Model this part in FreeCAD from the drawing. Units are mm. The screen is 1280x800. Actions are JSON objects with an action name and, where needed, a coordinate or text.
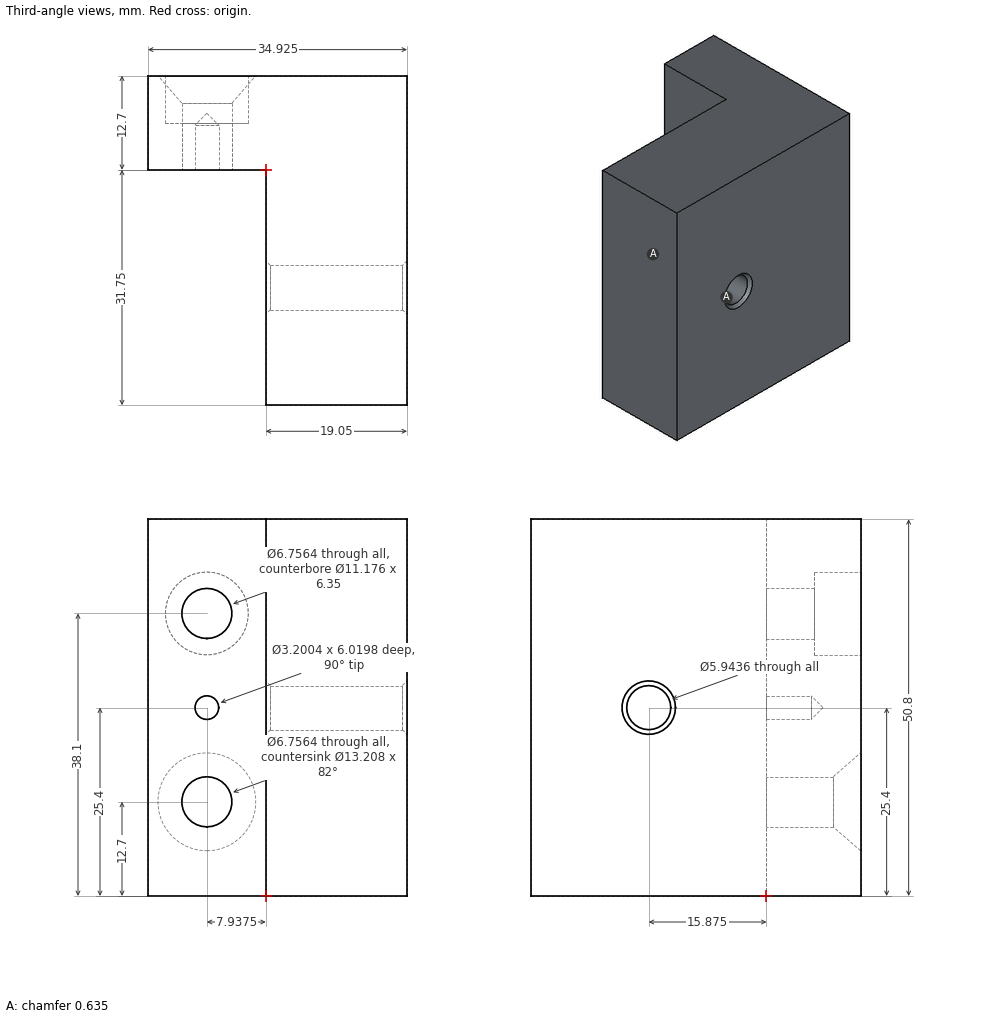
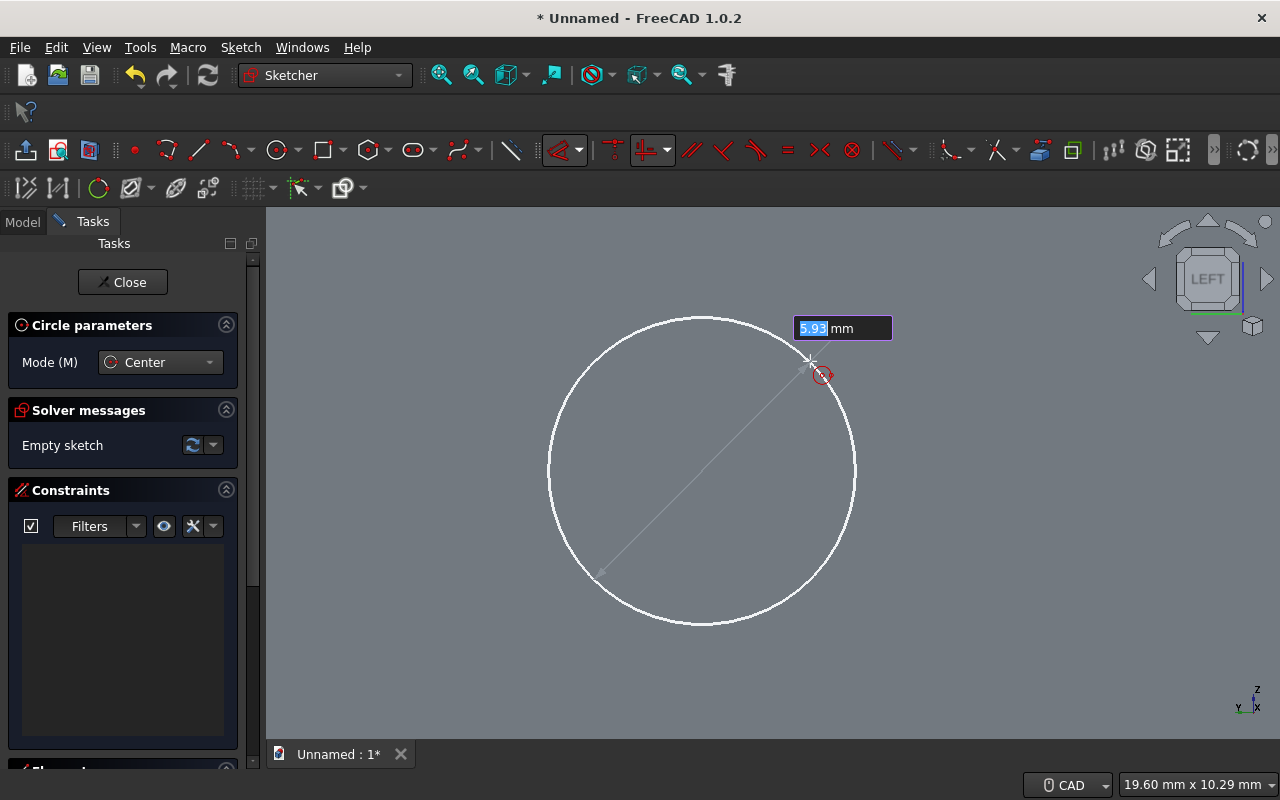
{"action": "type", "text": "5.9436"}
{"action": "key", "text": "Return"}
{"action": "key", "text": "Escape"}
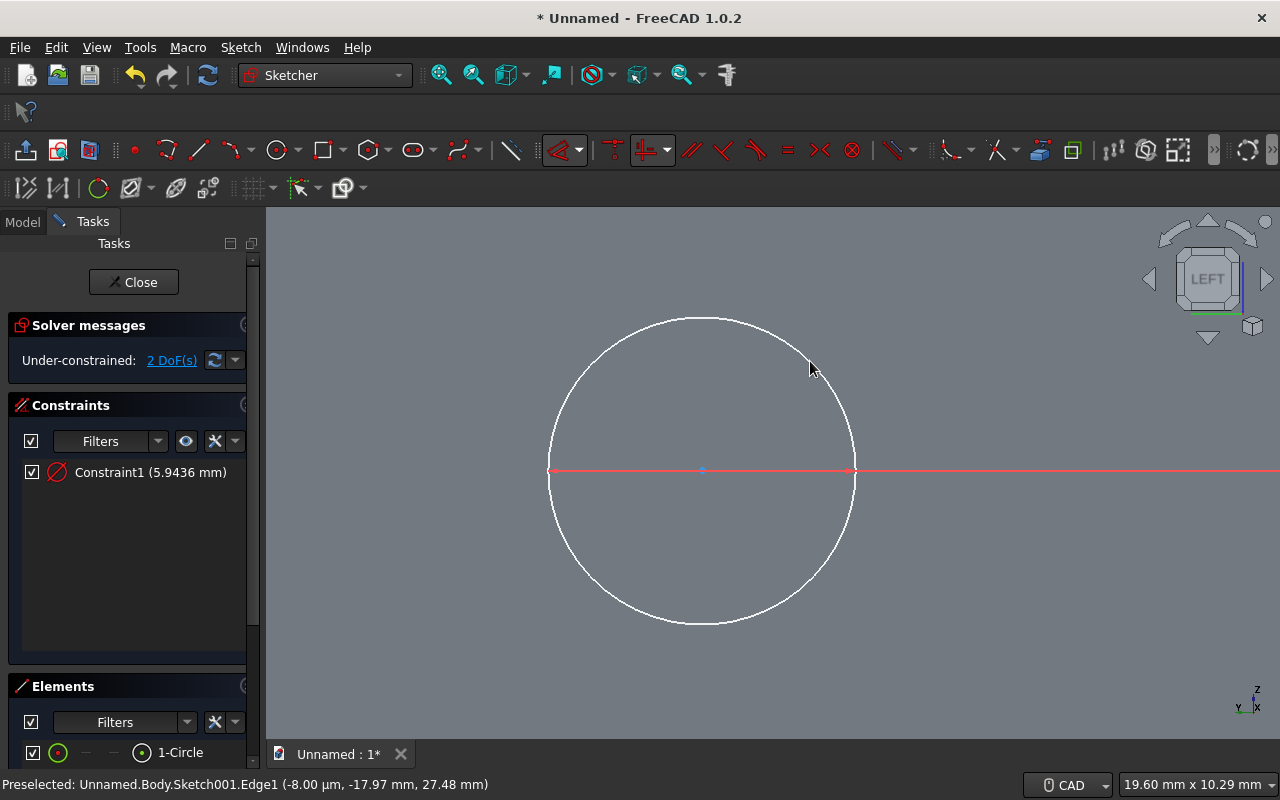
{"action": "left_click", "coordinate": [702, 471]}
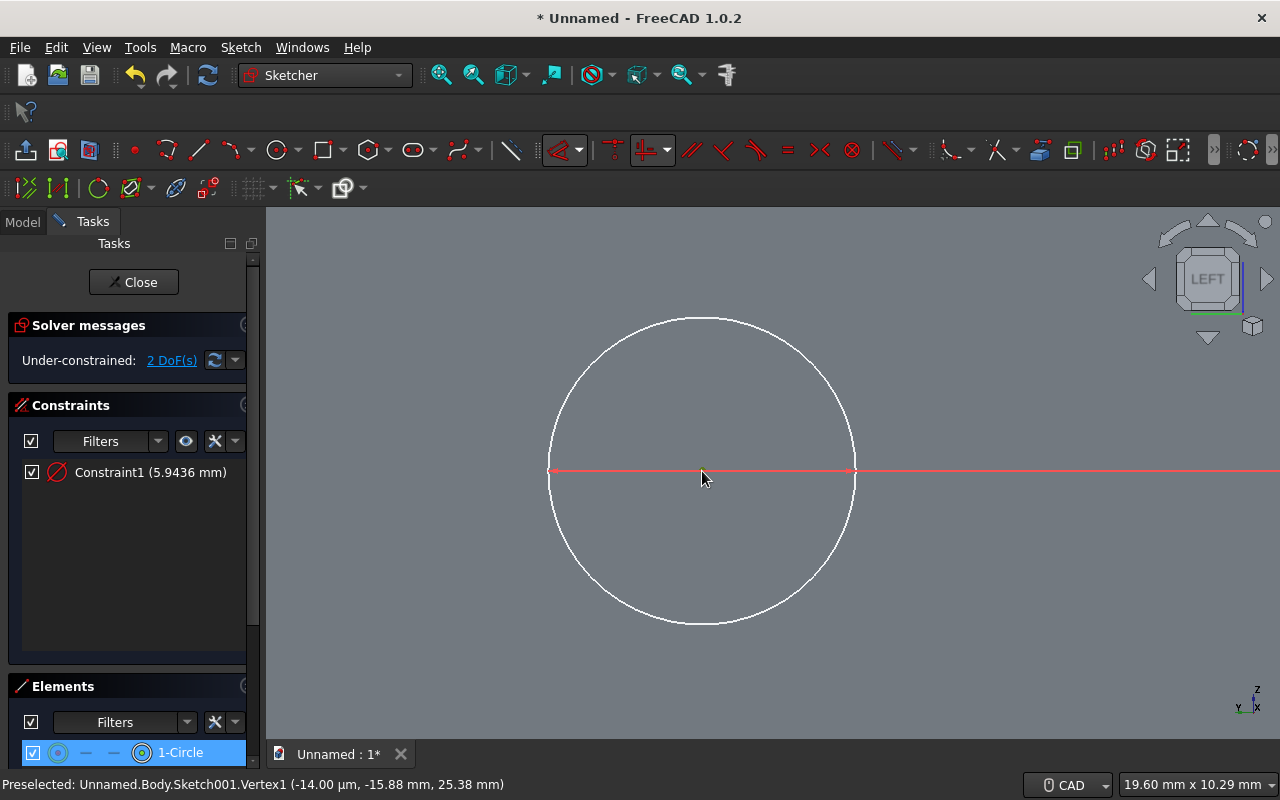
{"action": "left_click", "coordinate": [582, 150]}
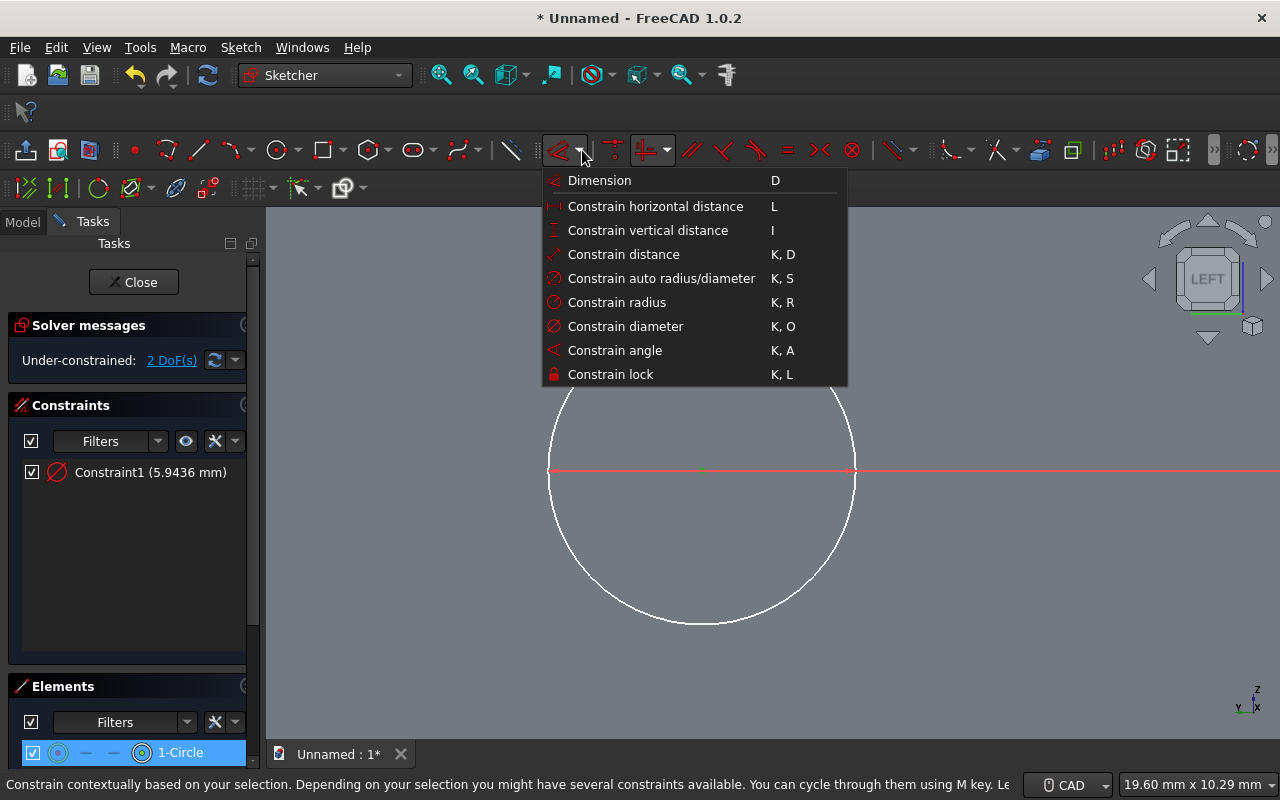
{"action": "left_click", "coordinate": [695, 230]}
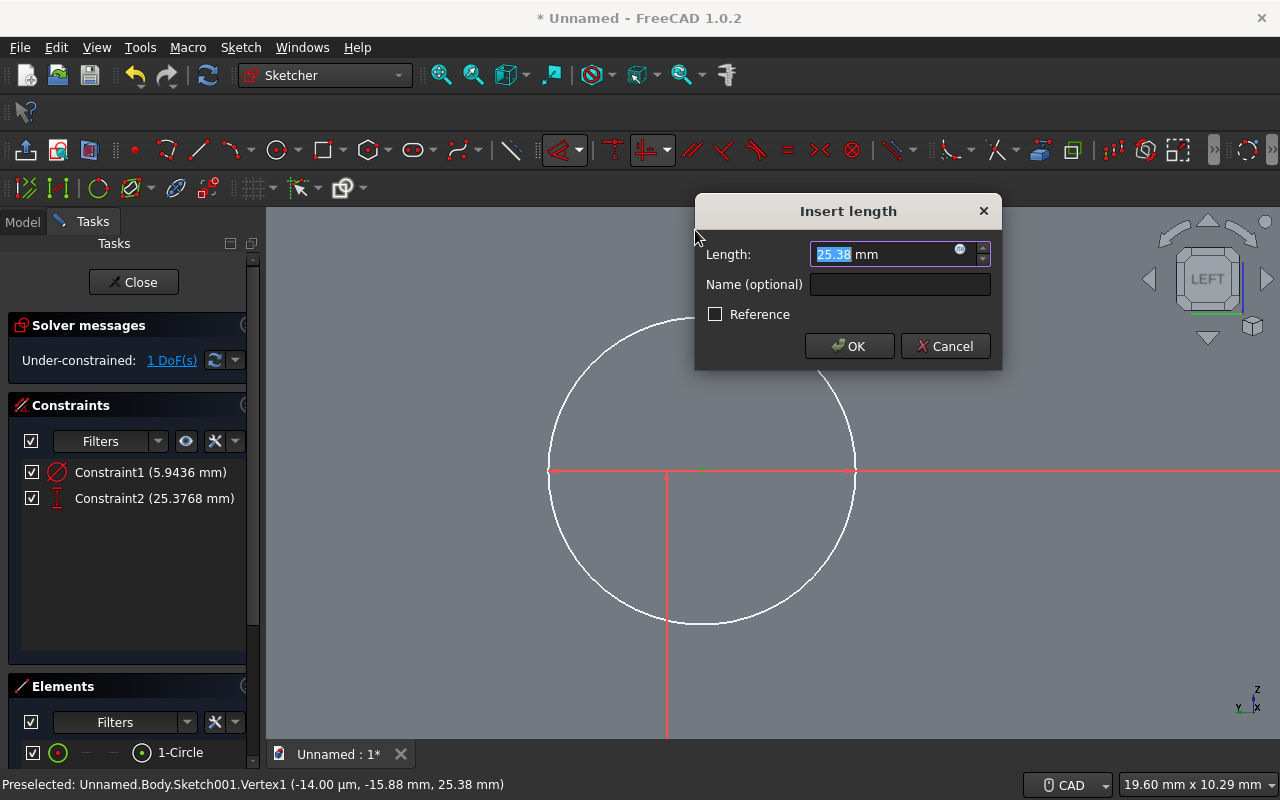
{"action": "type", "text": "25.4"}
{"action": "key", "text": "Return"}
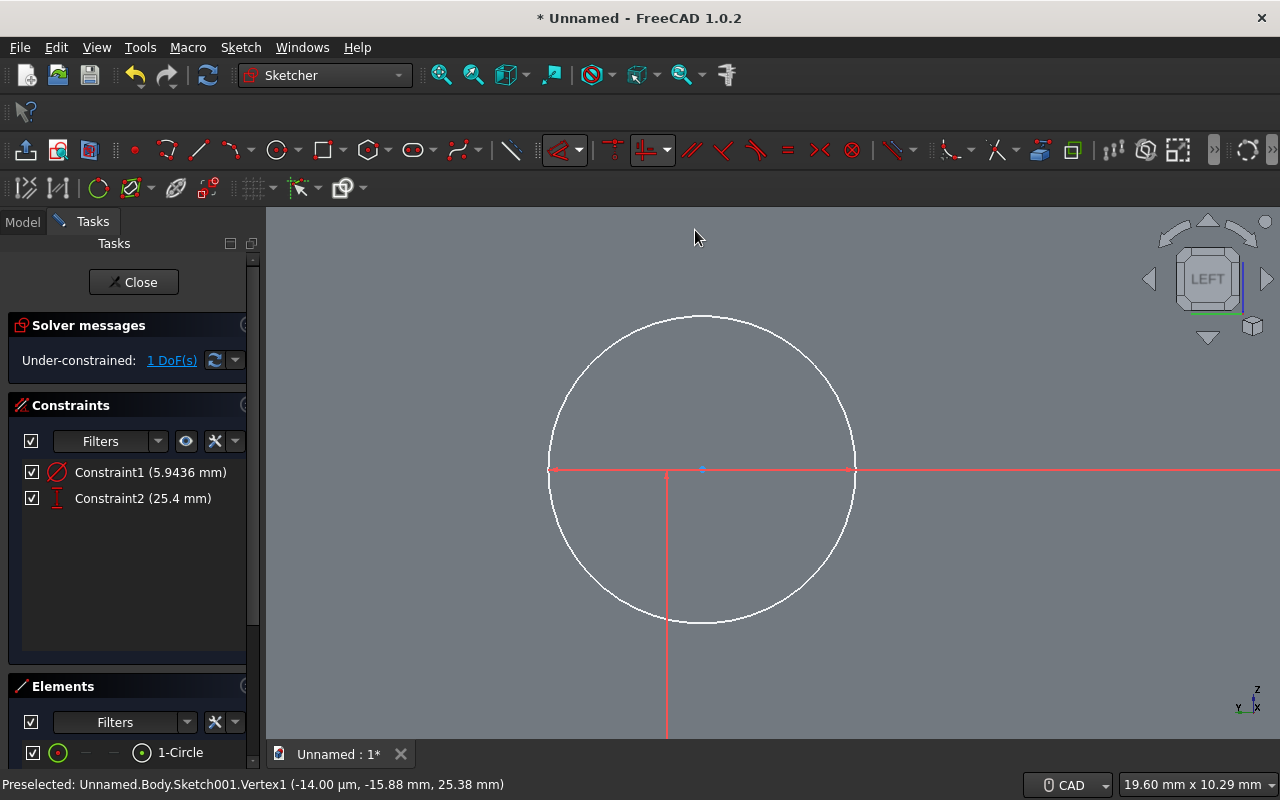
{"action": "left_click", "coordinate": [702, 470]}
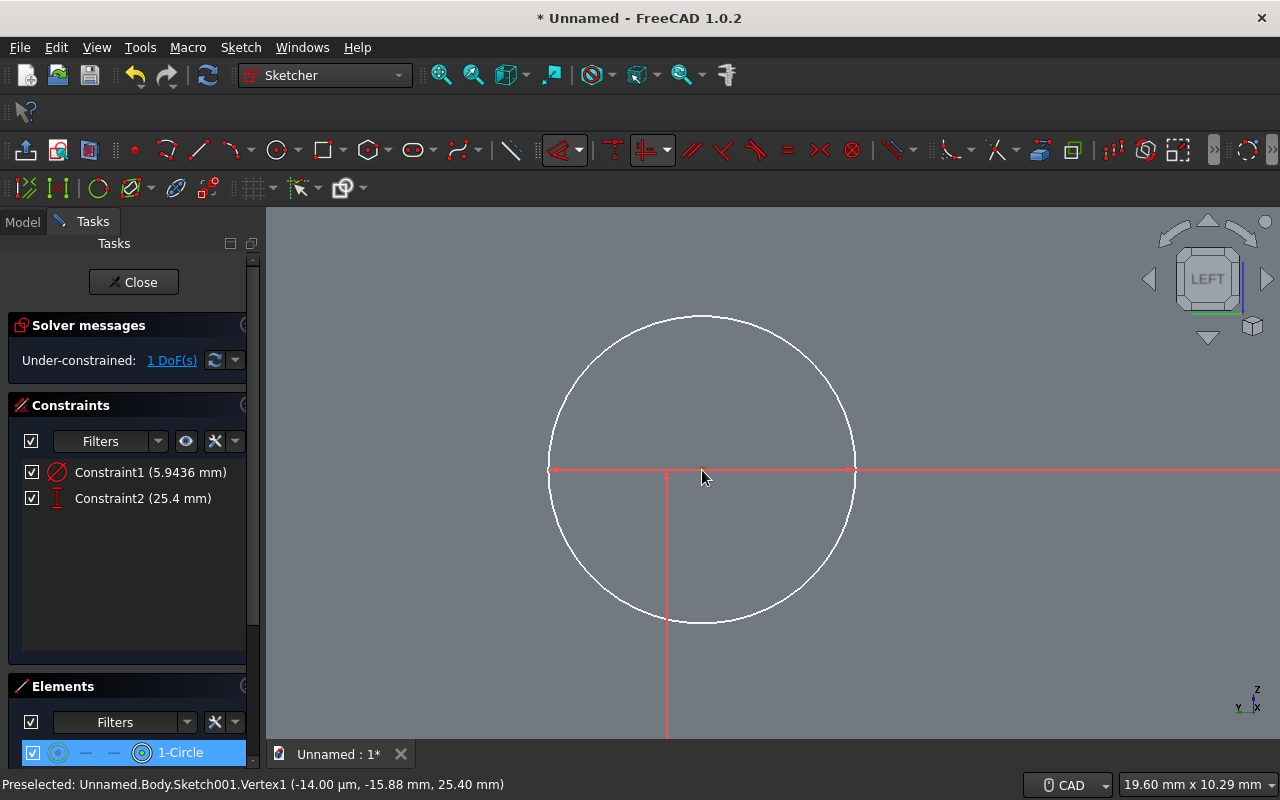
{"action": "key", "text": "l"}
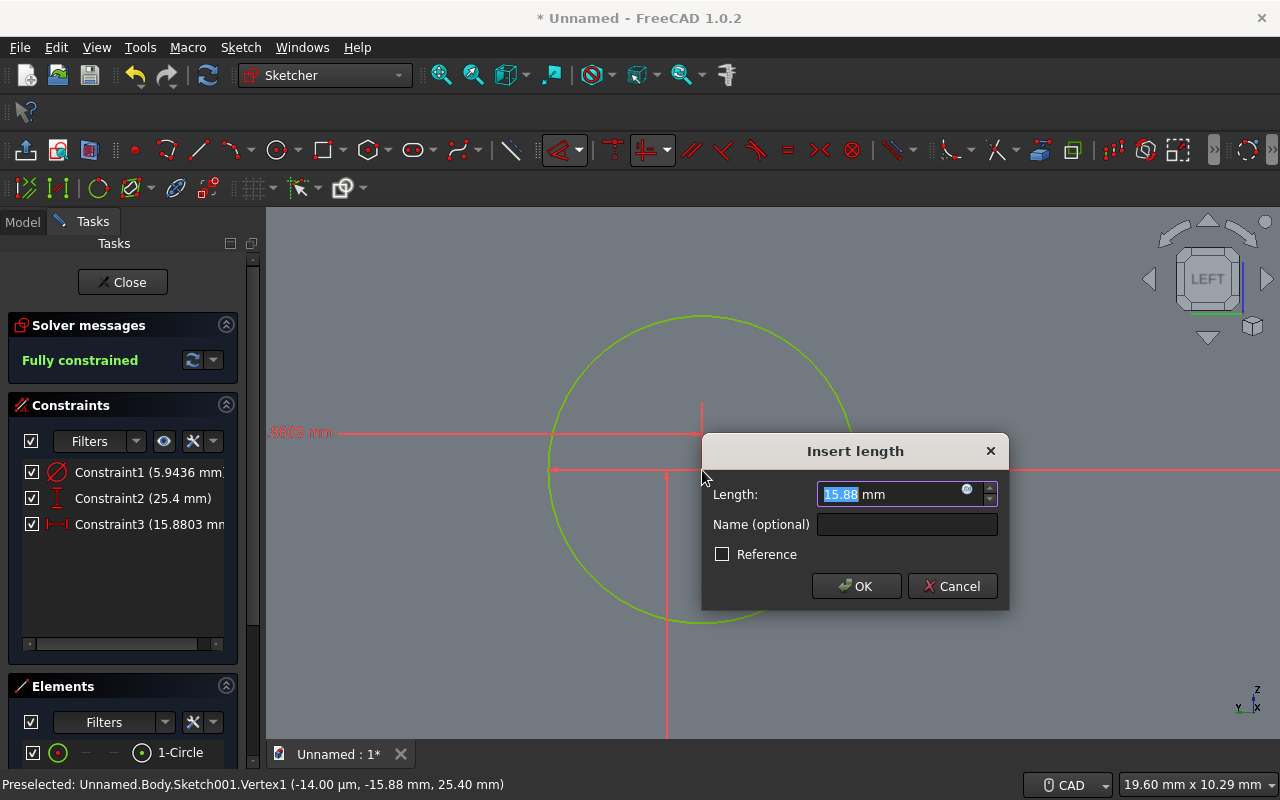
{"action": "type", "text": "15.875"}
{"action": "key", "text": "Return"}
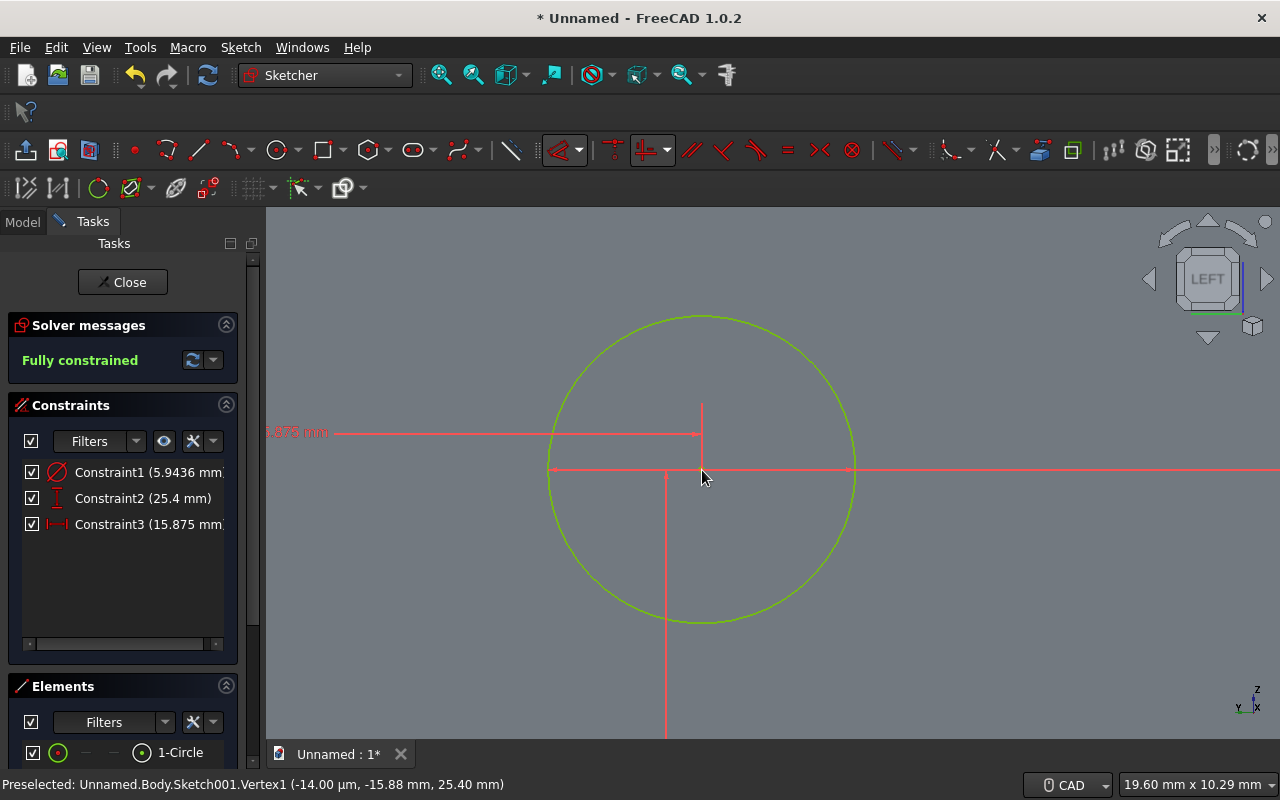
{"action": "left_click", "coordinate": [123, 282]}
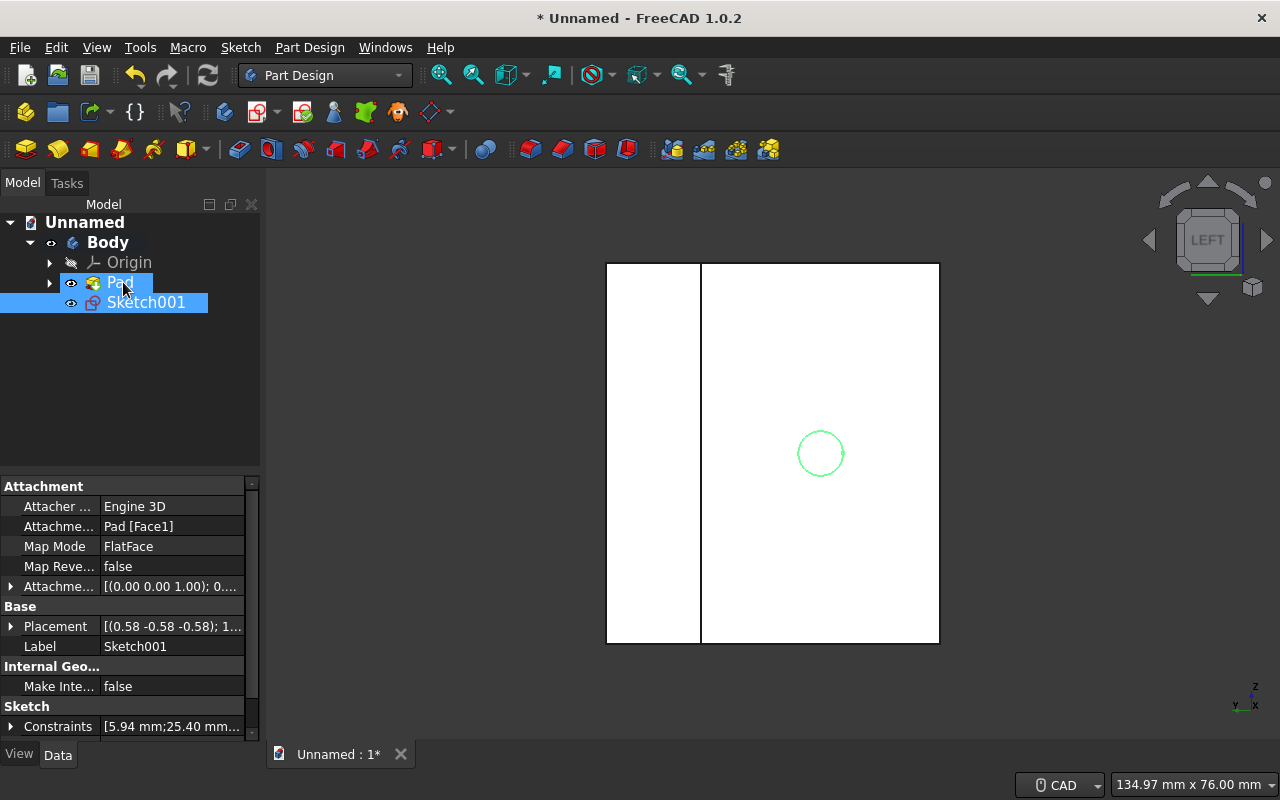
{"action": "left_click", "coordinate": [272, 150]}